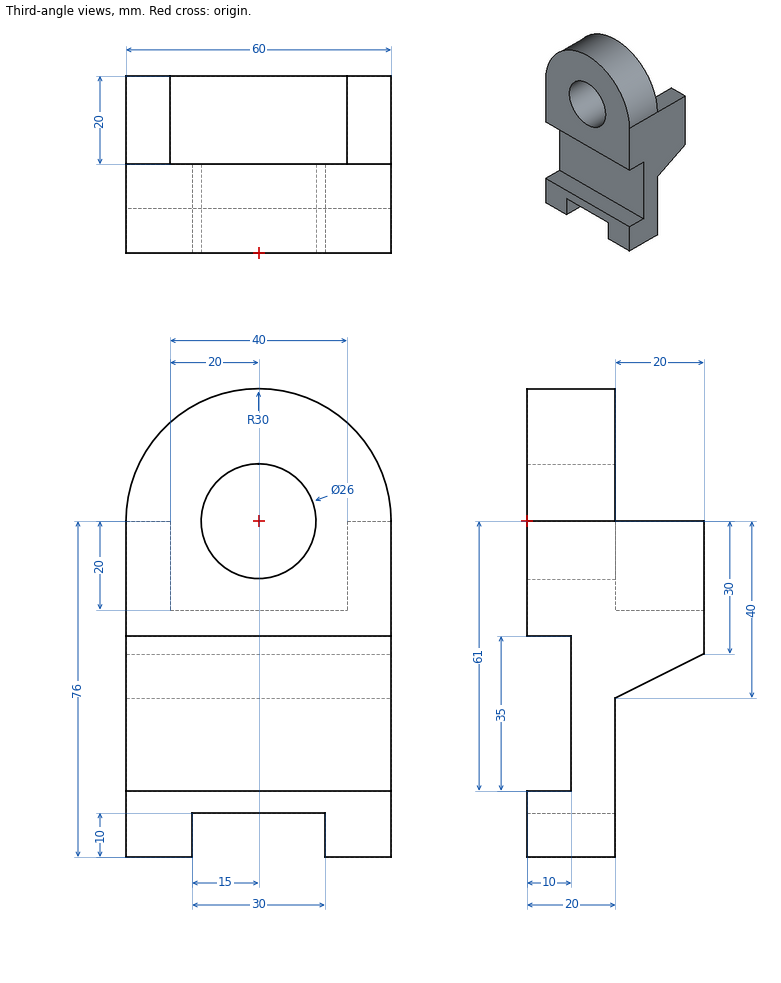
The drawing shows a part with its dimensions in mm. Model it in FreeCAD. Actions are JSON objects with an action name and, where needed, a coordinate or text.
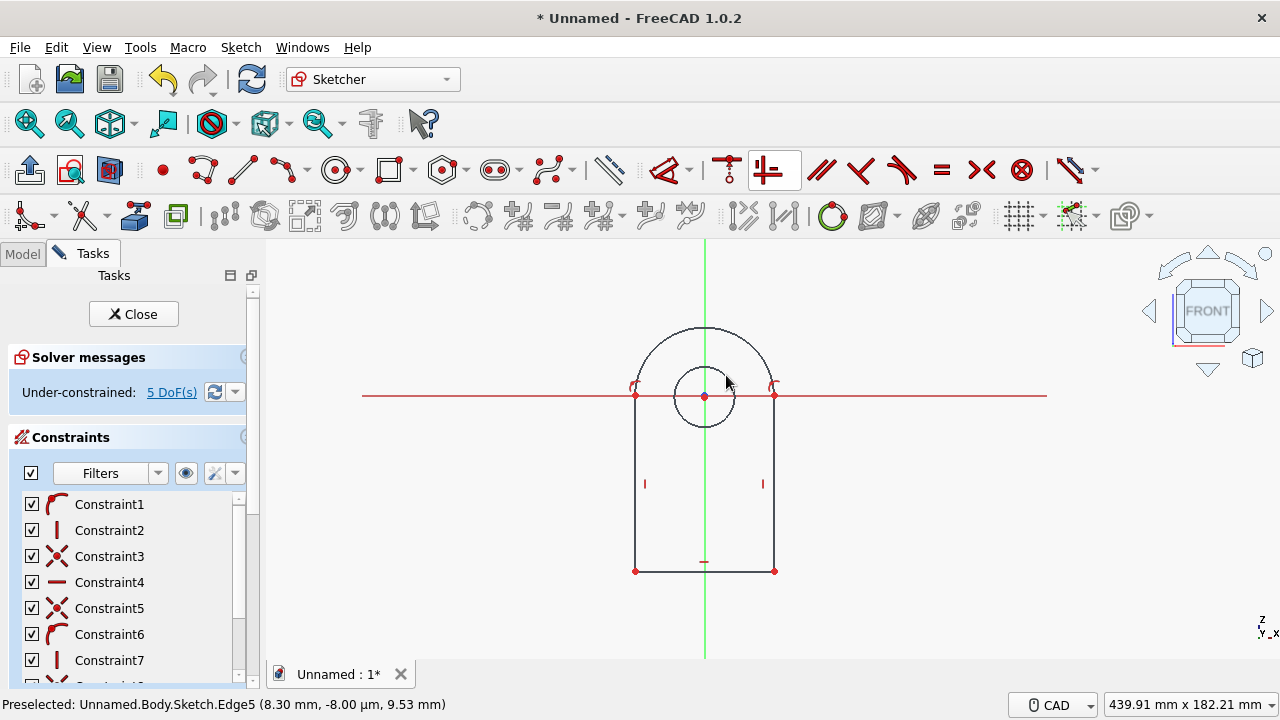
{"action": "scroll", "coordinate": [705, 396], "scroll_direction": "up", "scroll_amount": 2}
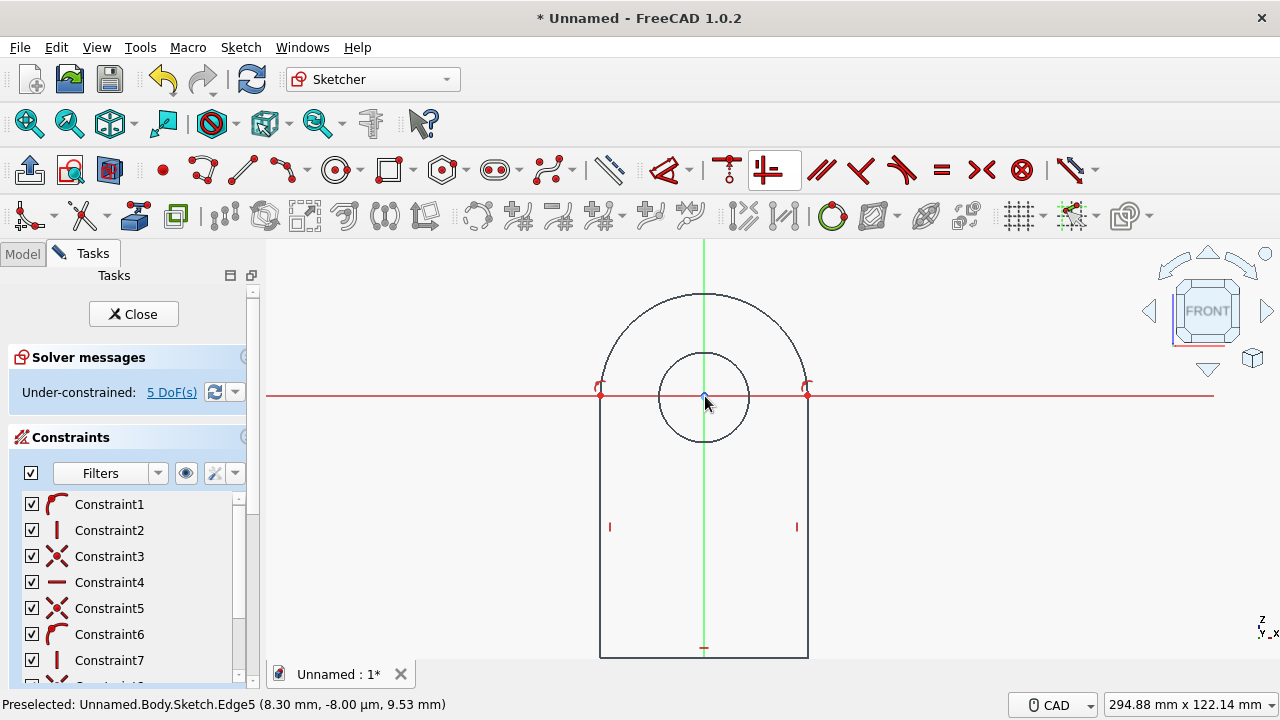
{"action": "left_click_drag", "start_coordinate": [694, 386], "coordinate": [714, 407]}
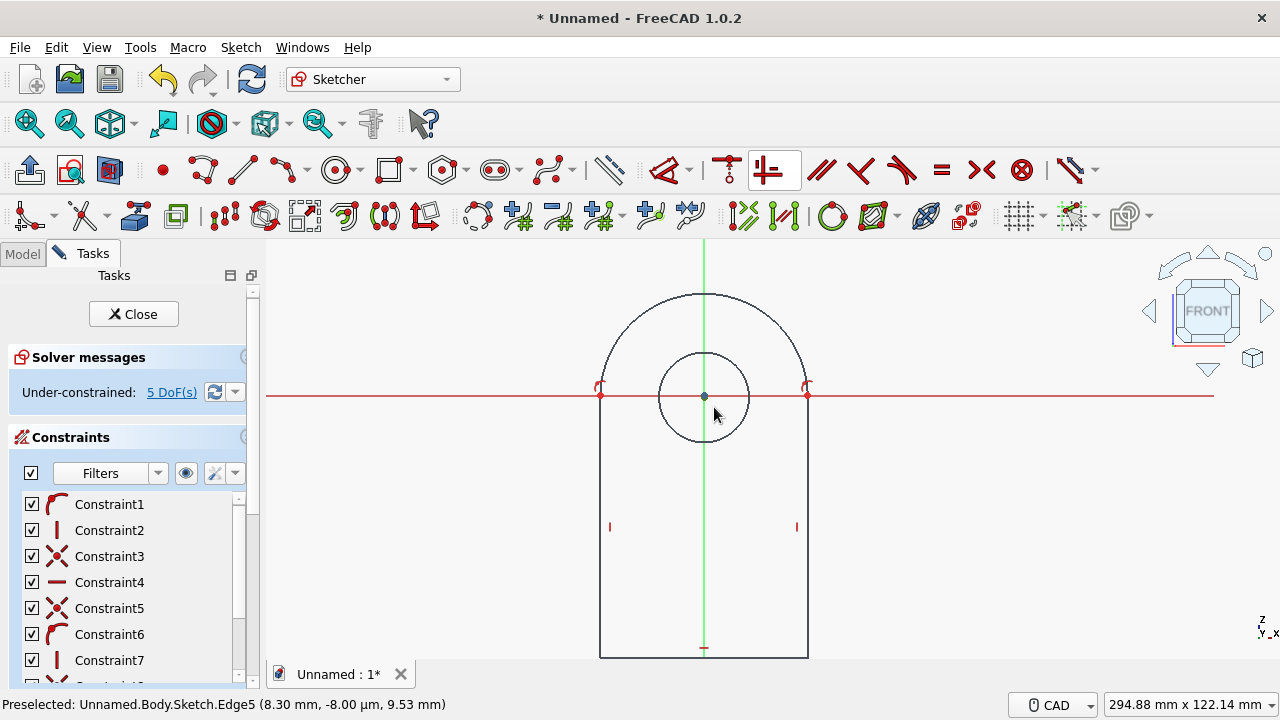
{"action": "key", "text": "c"}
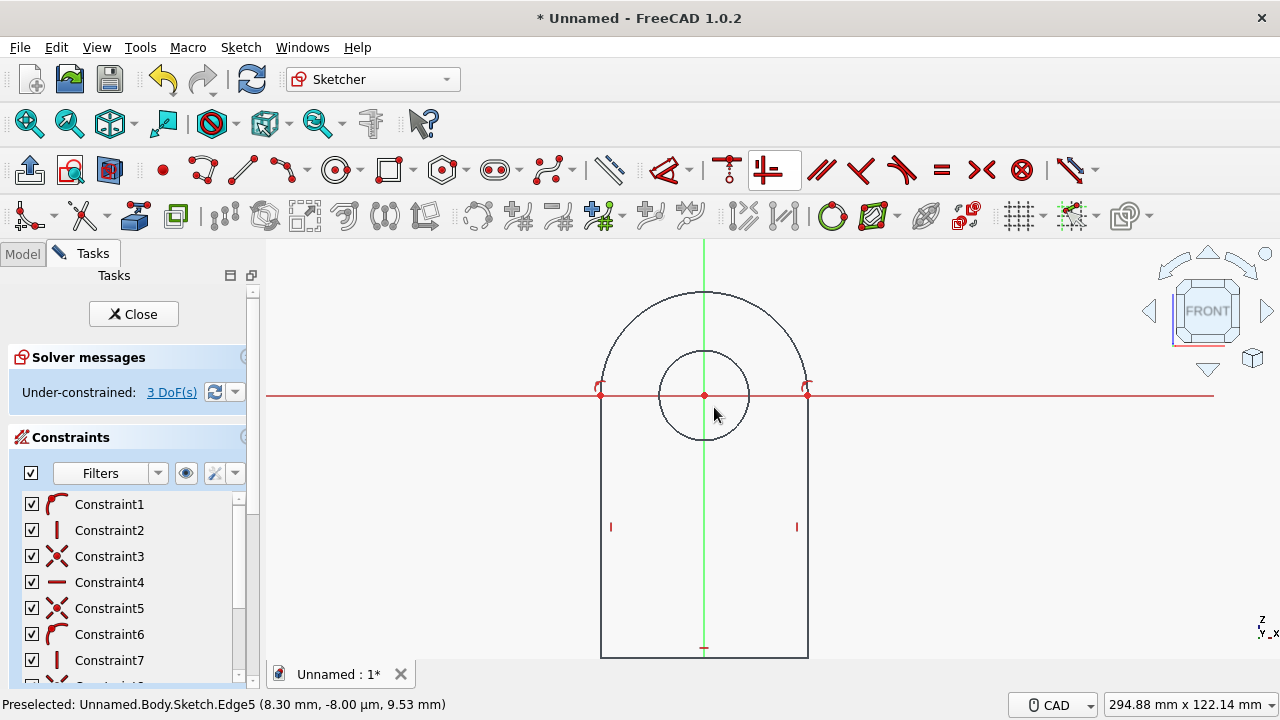
{"action": "left_click", "coordinate": [765, 312]}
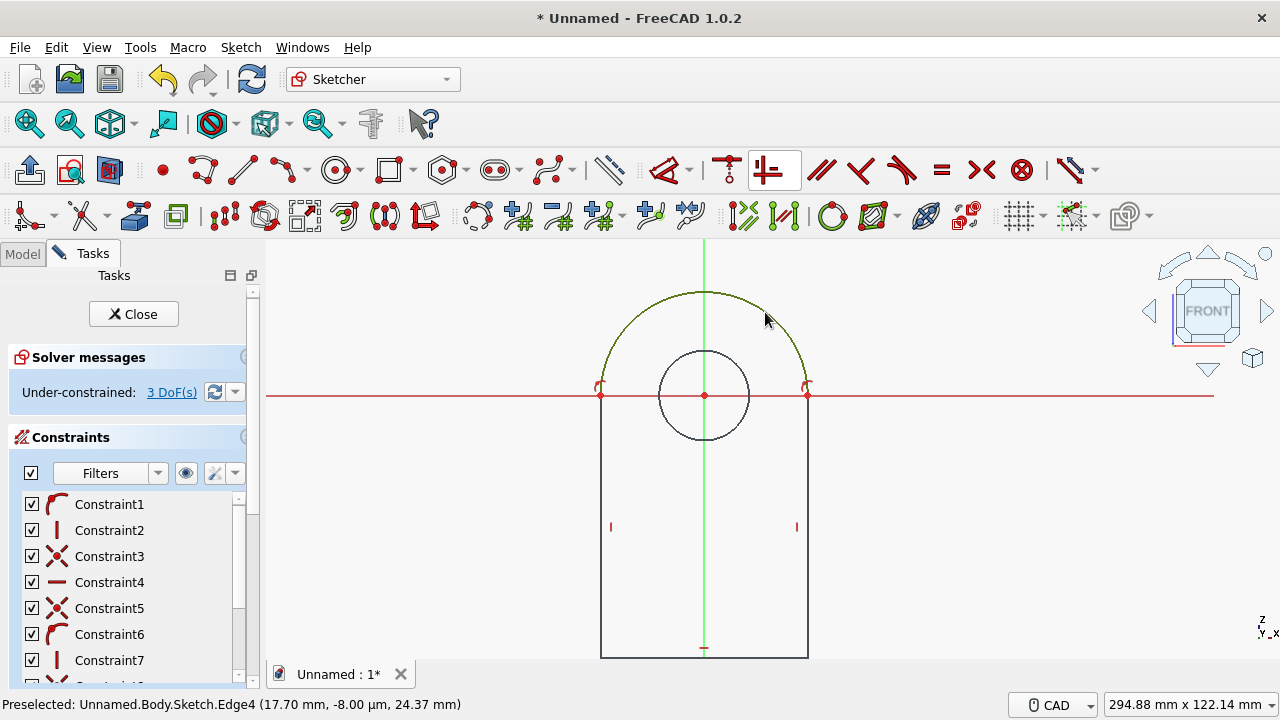
{"action": "left_click", "coordinate": [692, 170]}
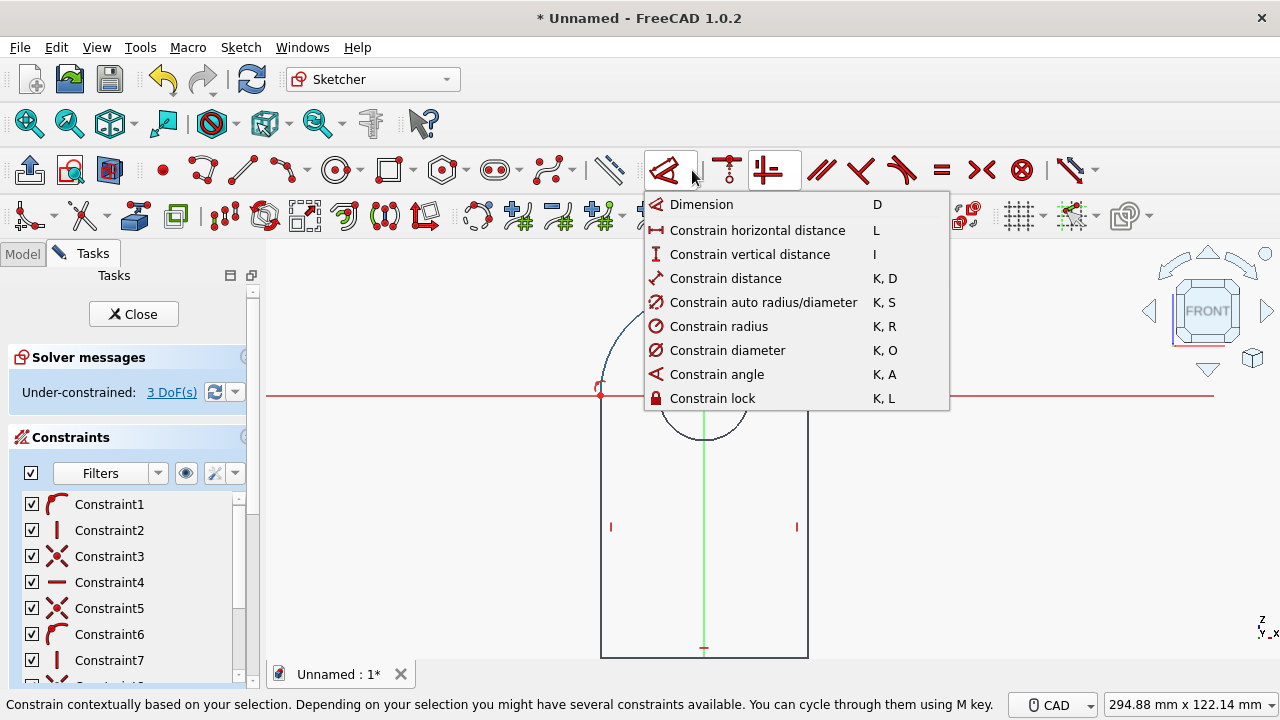
{"action": "left_click", "coordinate": [797, 326]}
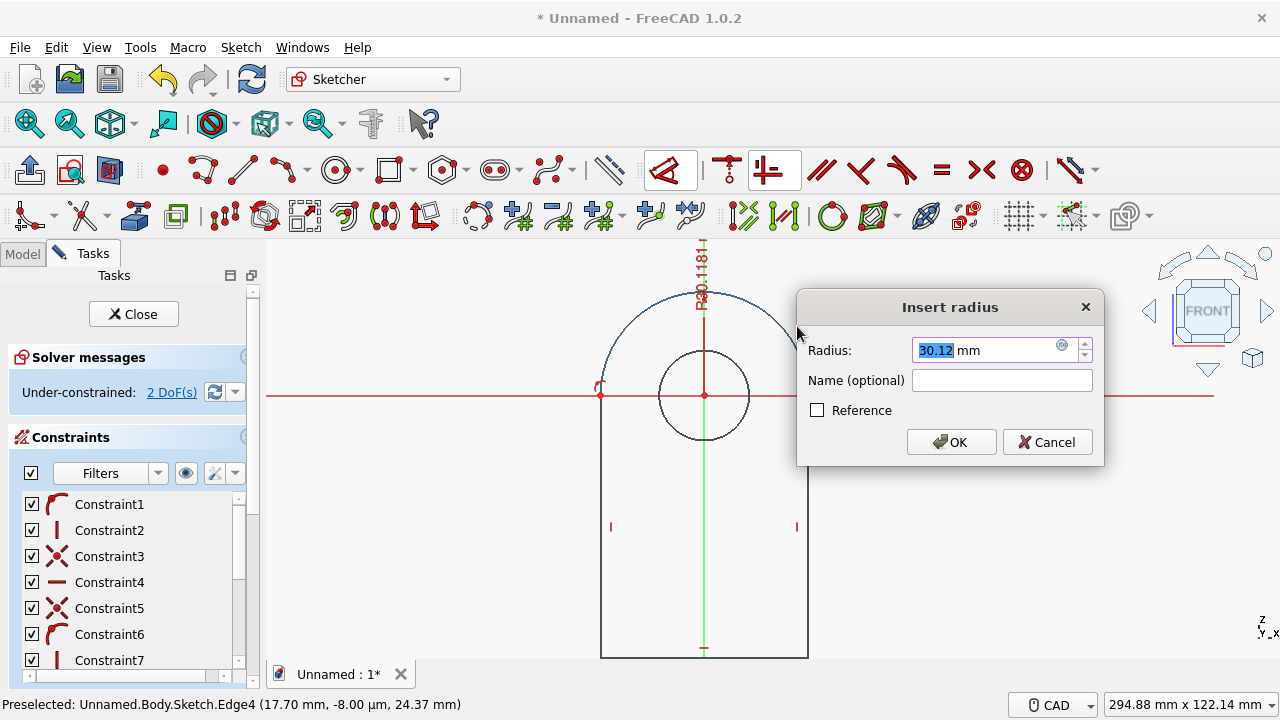
{"action": "type", "text": "30"}
{"action": "key", "text": "Return"}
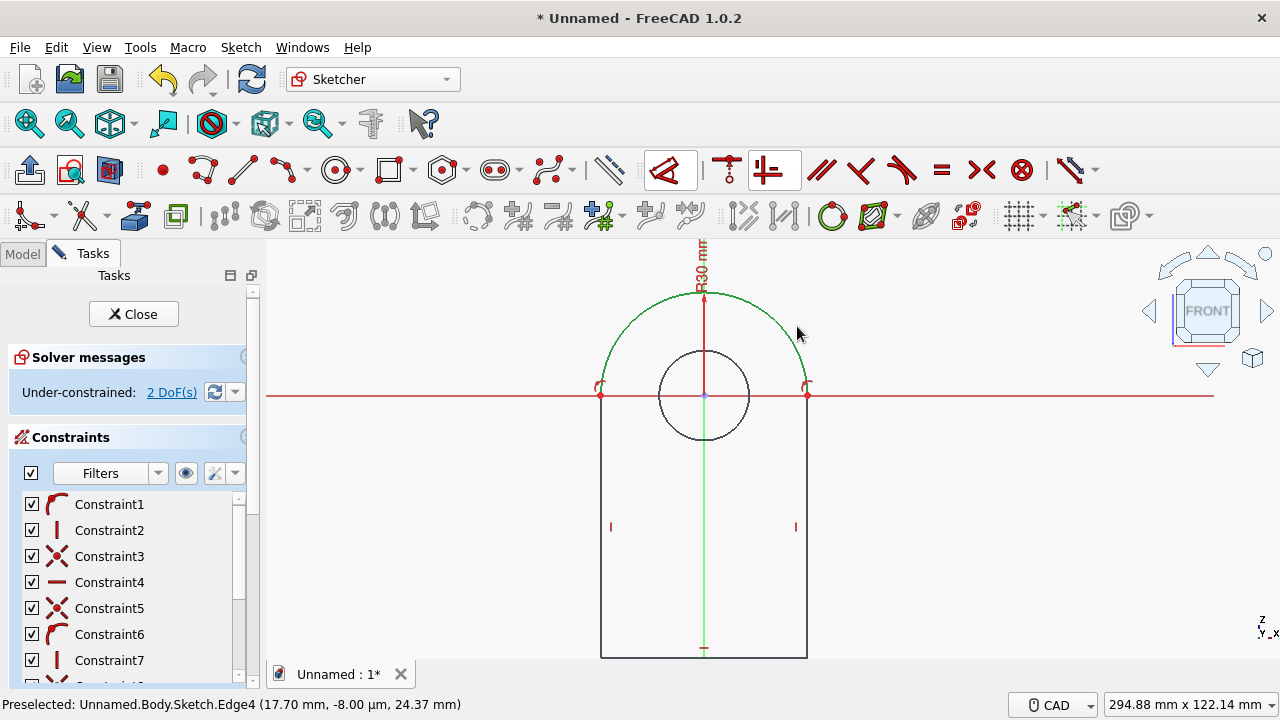
{"action": "left_click", "coordinate": [736, 364]}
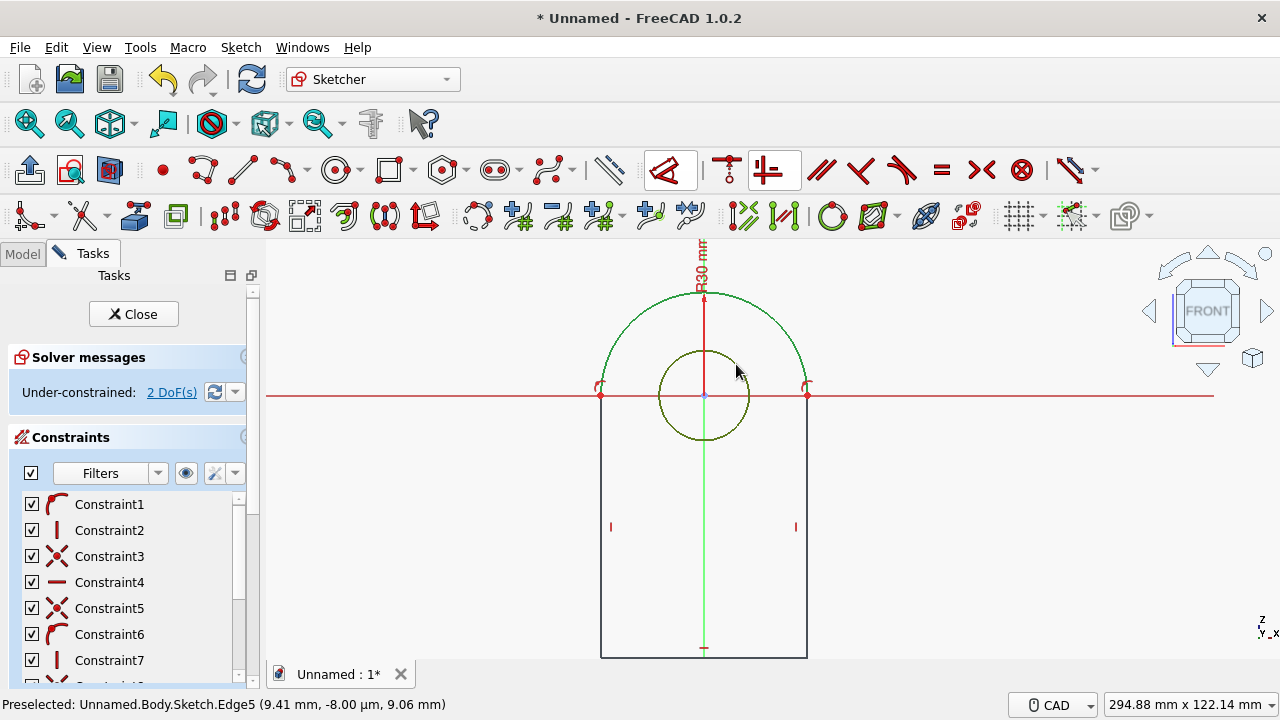
{"action": "left_click", "coordinate": [692, 170]}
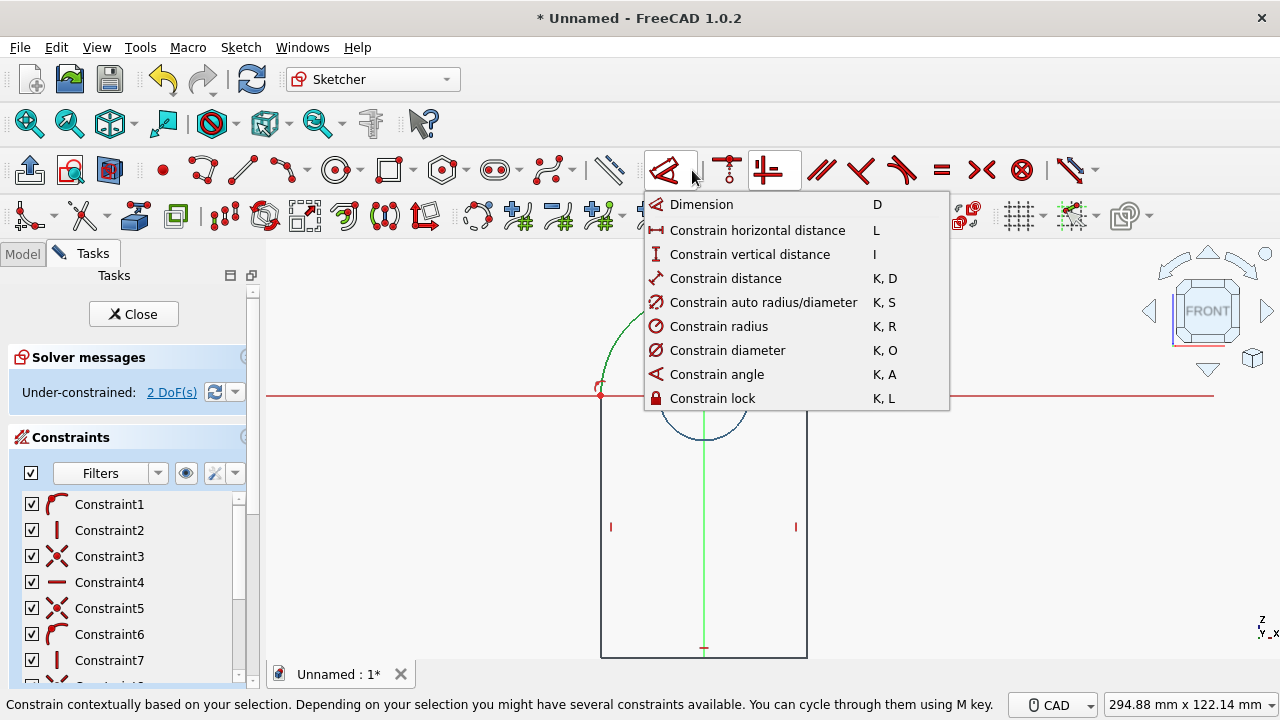
{"action": "left_click", "coordinate": [797, 350]}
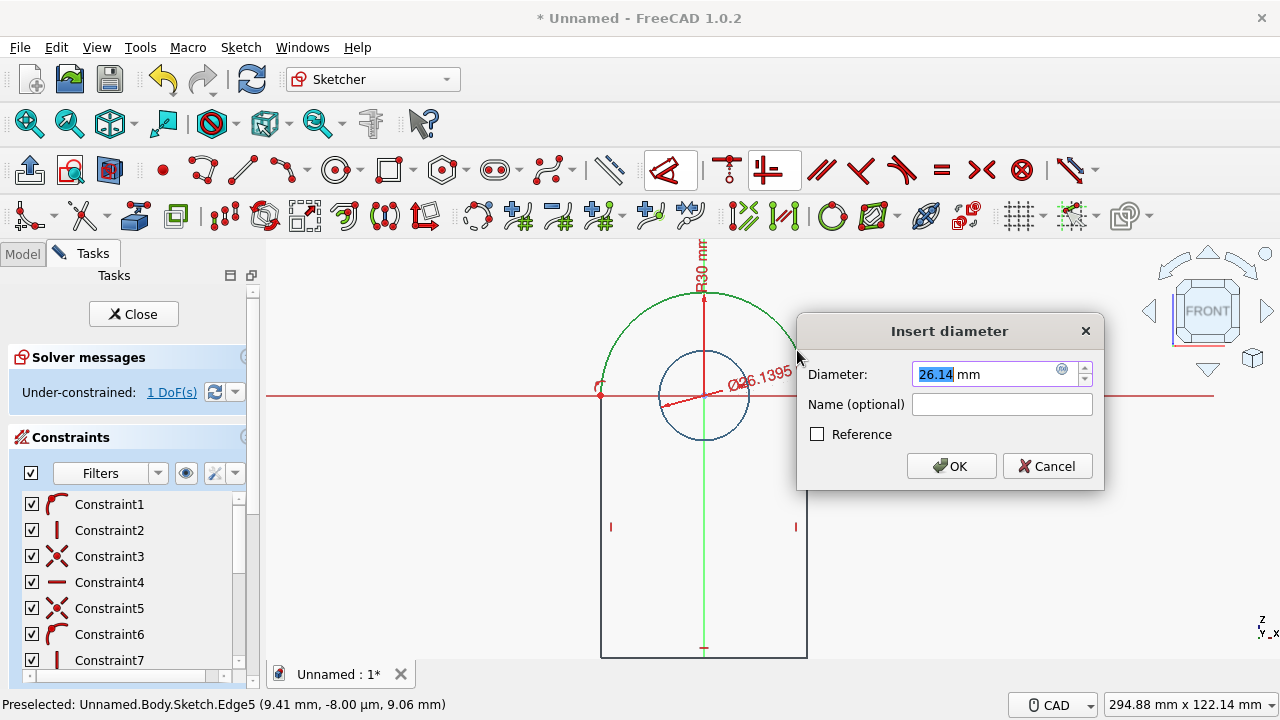
{"action": "type", "text": "26"}
{"action": "key", "text": "Return"}